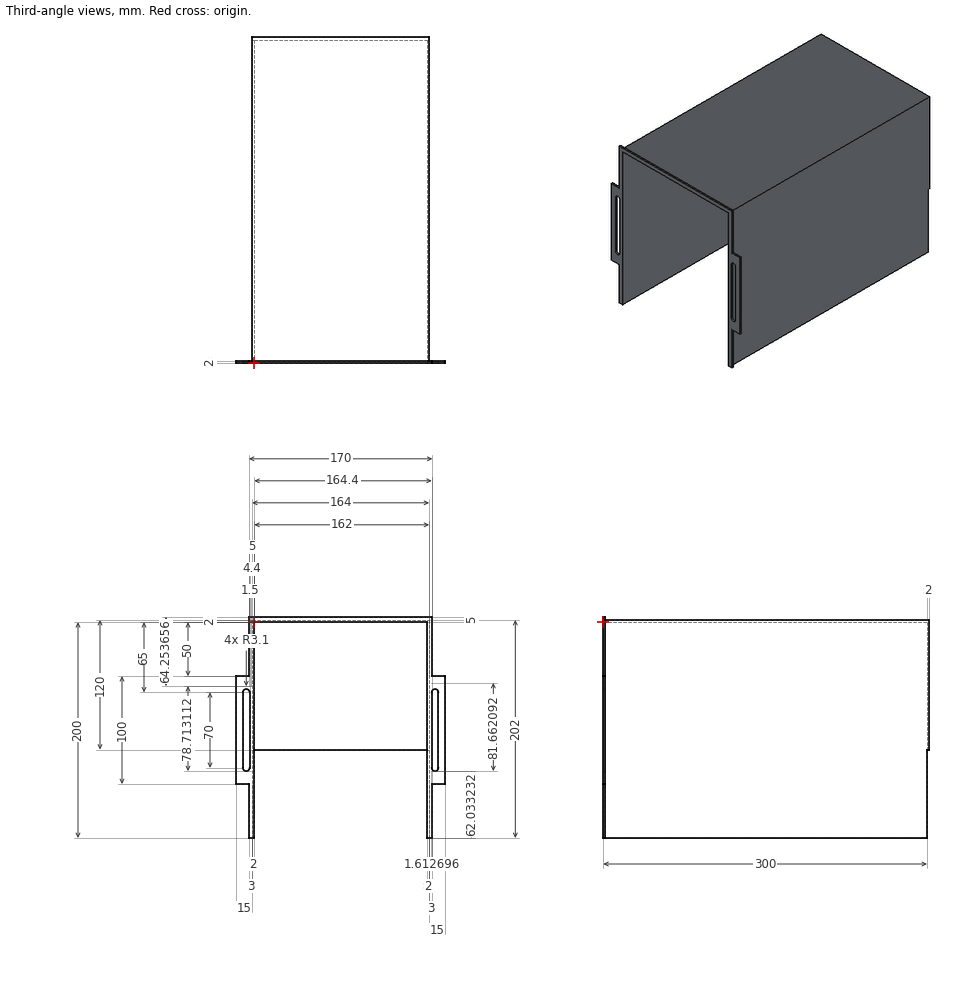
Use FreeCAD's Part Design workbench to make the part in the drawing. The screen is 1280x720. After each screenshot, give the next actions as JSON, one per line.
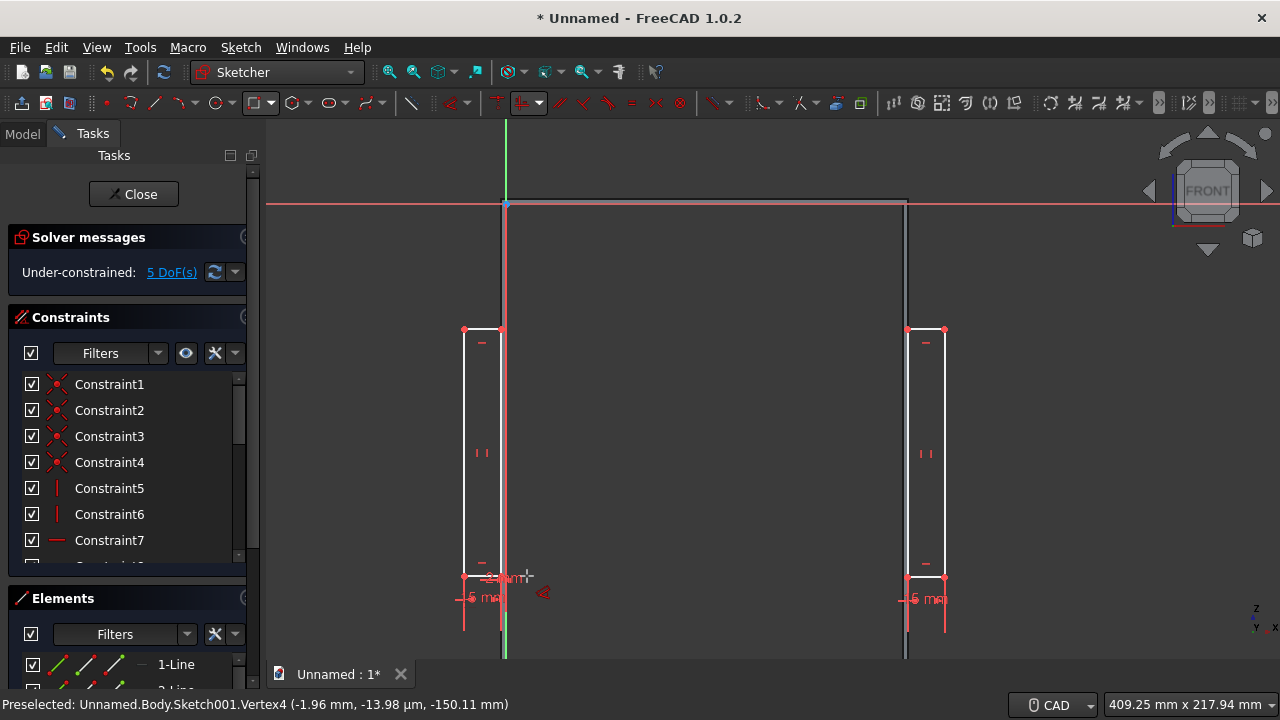
{"action": "left_click", "coordinate": [464, 404]}
{"action": "left_click", "coordinate": [430, 453]}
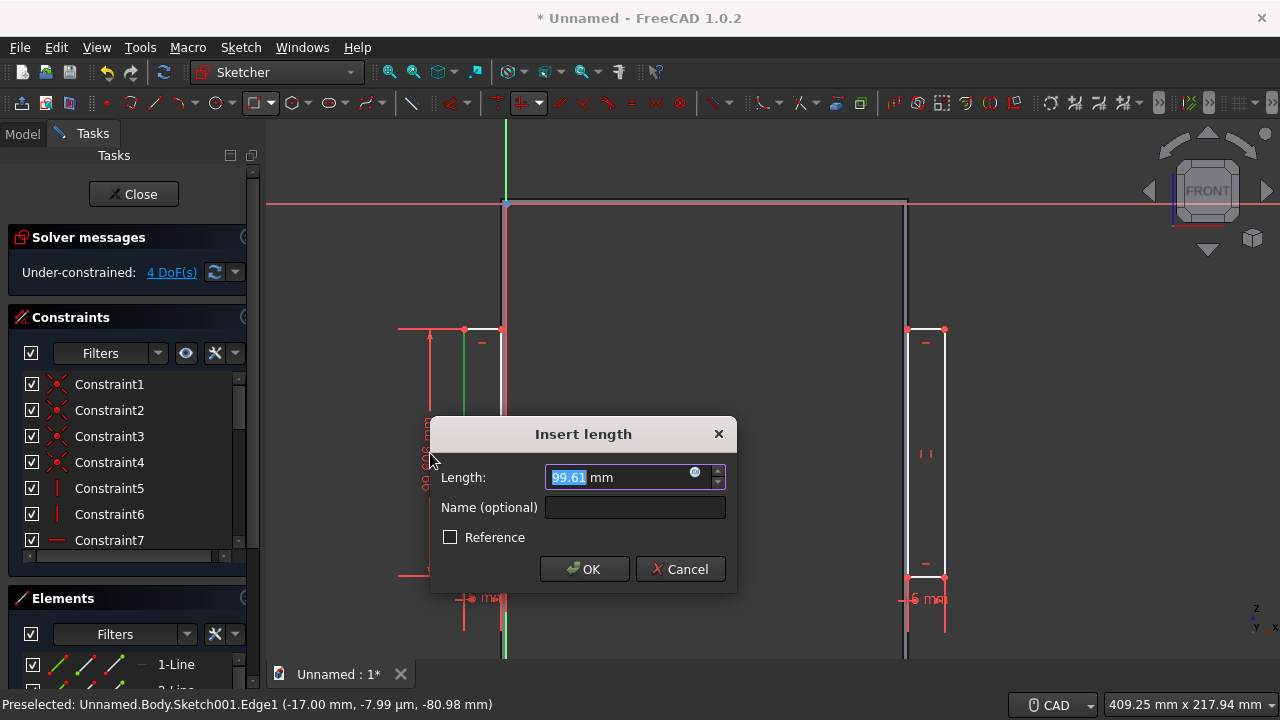
{"action": "type", "text": "100"}
{"action": "key", "text": "Return"}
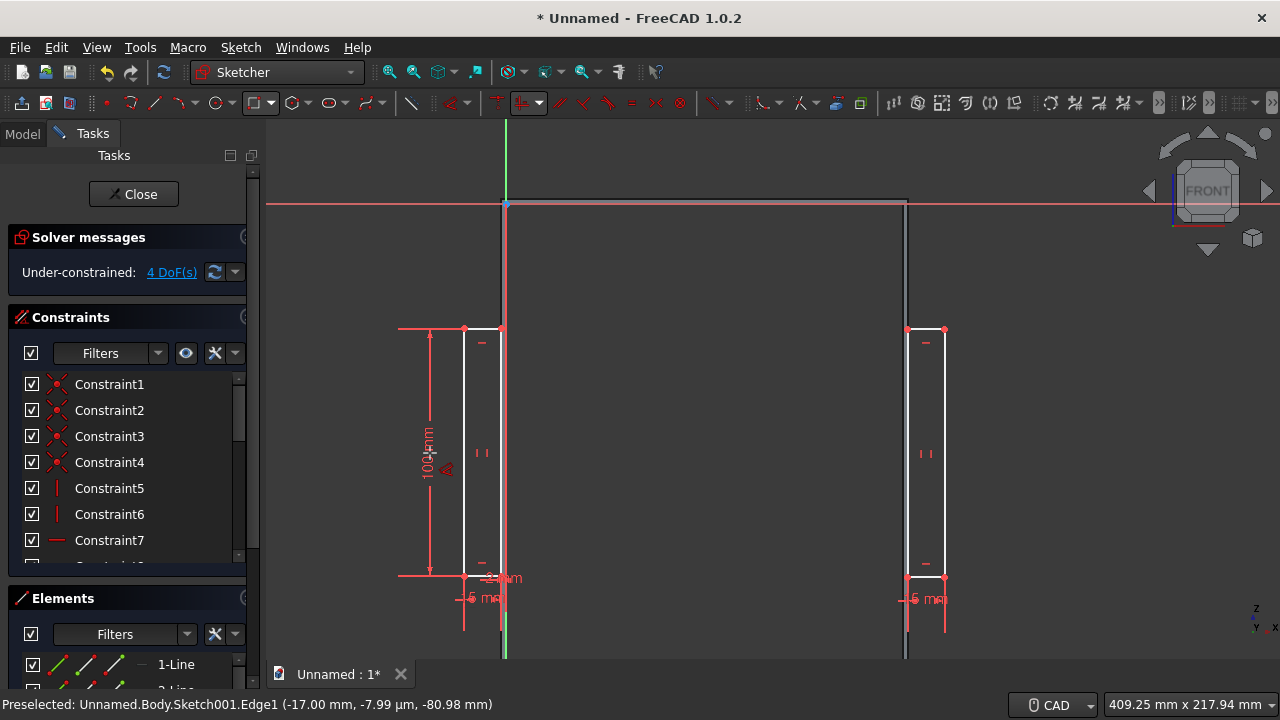
{"action": "left_click", "coordinate": [908, 404]}
{"action": "left_click", "coordinate": [874, 453]}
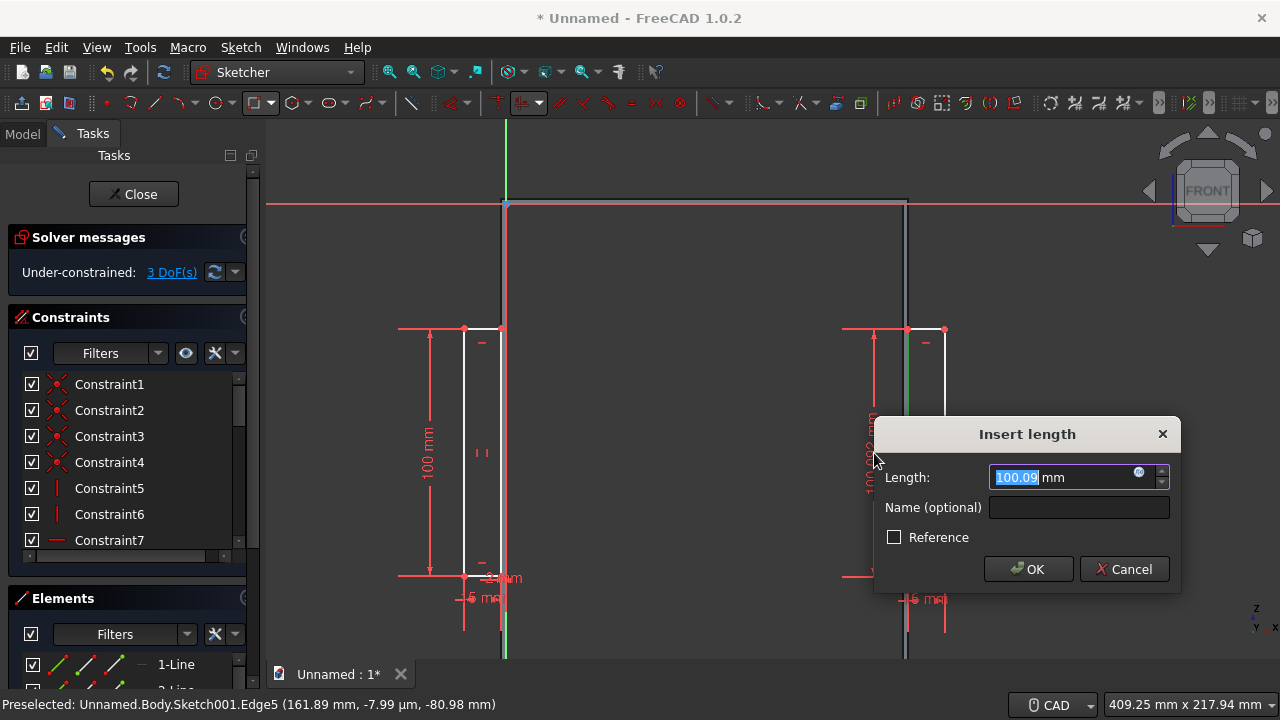
{"action": "type", "text": "100"}
{"action": "key", "text": "Return"}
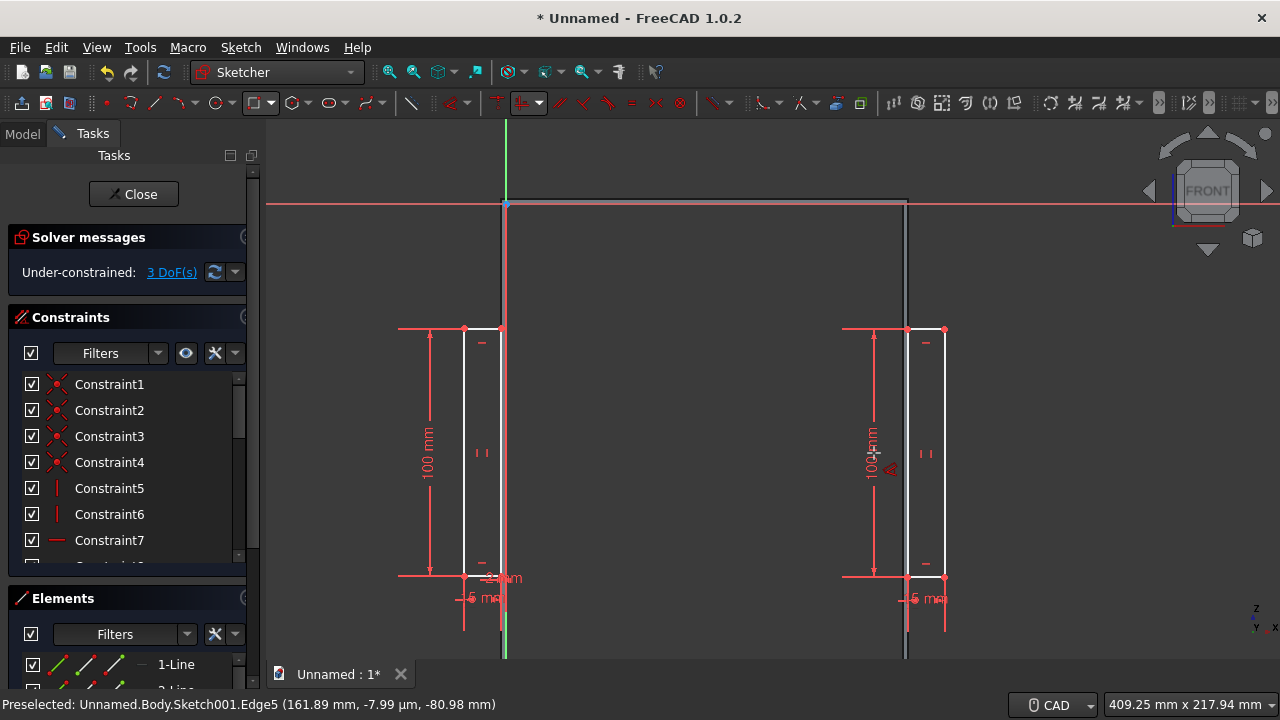
{"action": "left_click", "coordinate": [464, 329]}
{"action": "left_click", "coordinate": [430, 267]}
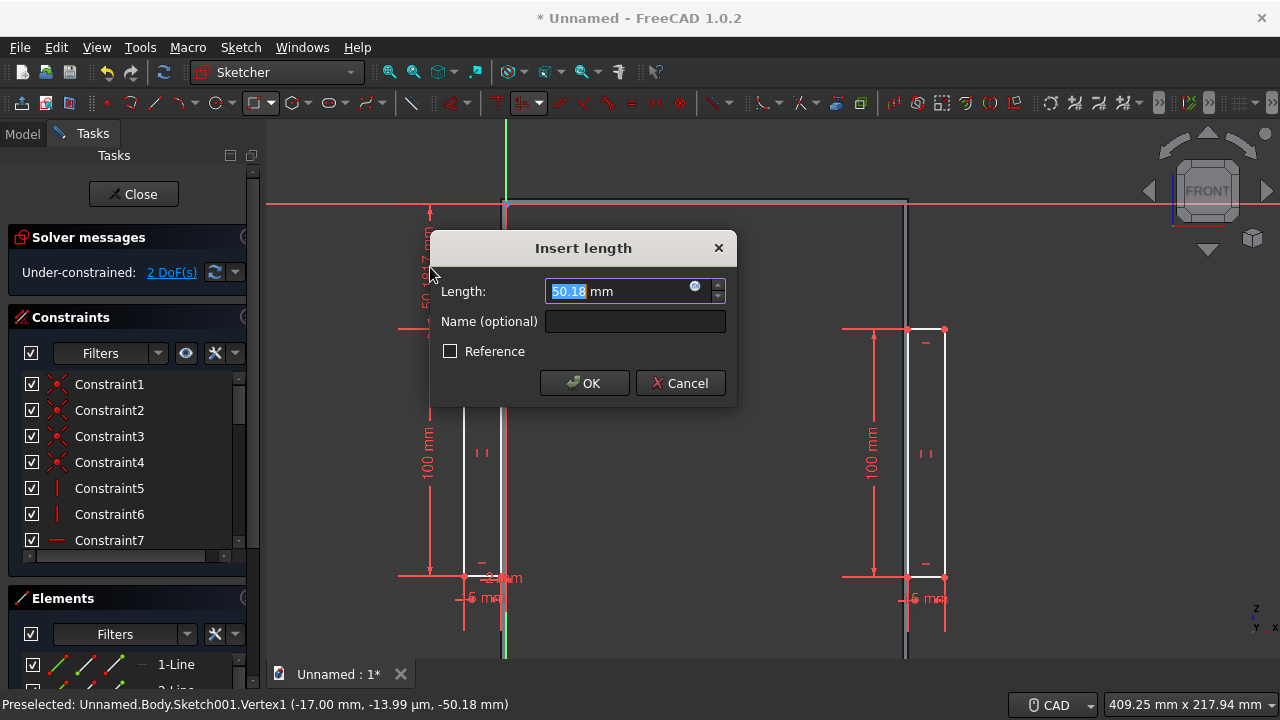
{"action": "type", "text": "50"}
{"action": "key", "text": "Return"}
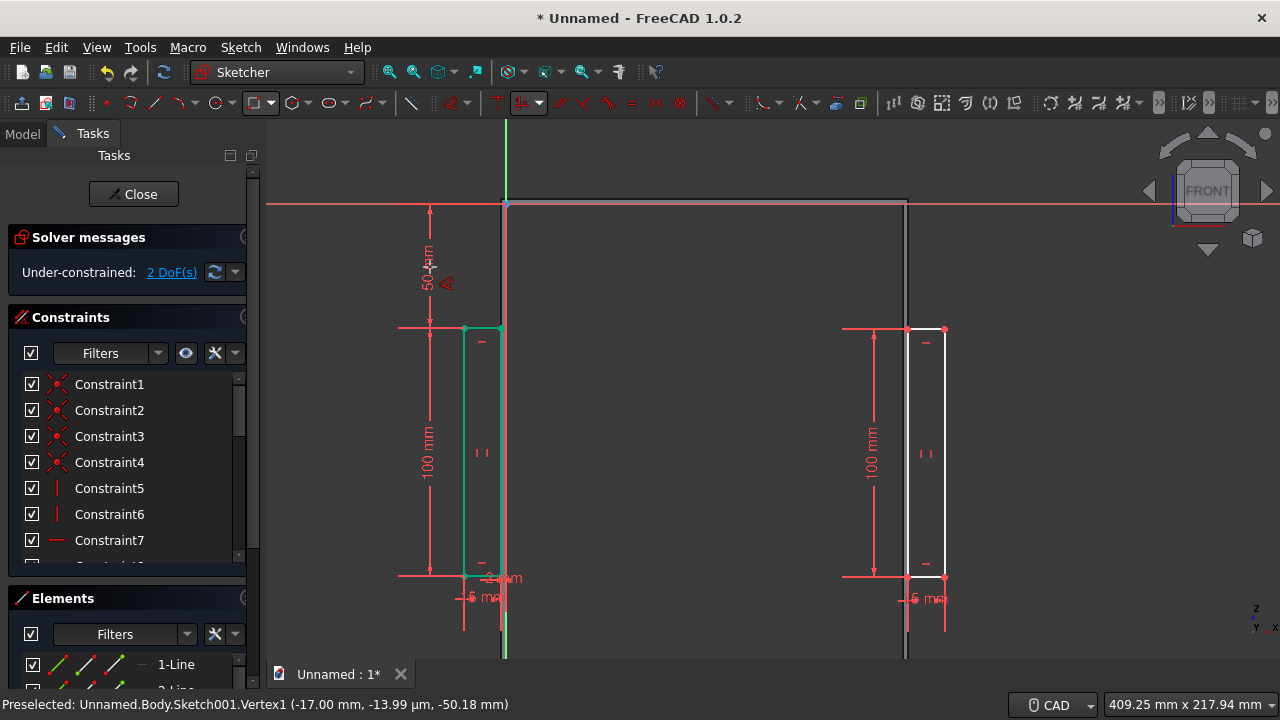
{"action": "left_click", "coordinate": [908, 329]}
{"action": "left_click", "coordinate": [942, 267]}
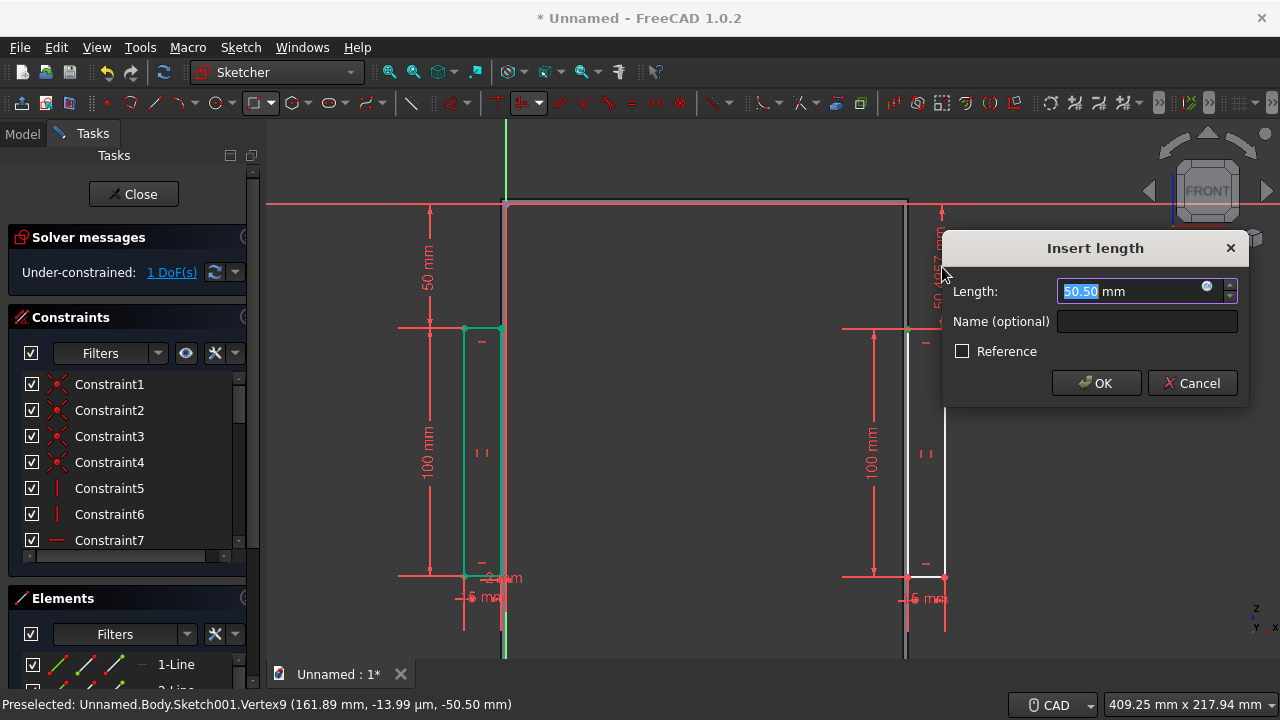
{"action": "type", "text": "50"}
{"action": "key", "text": "Return"}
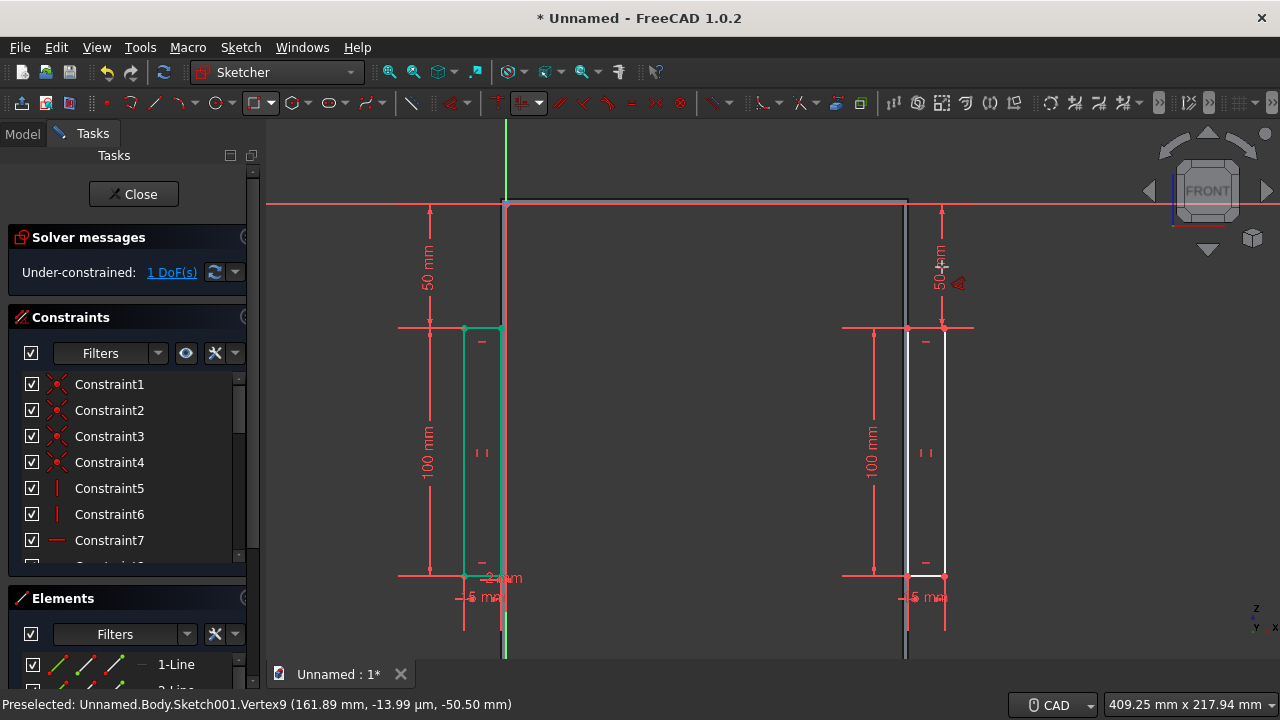
{"action": "left_click", "coordinate": [908, 328]}
{"action": "left_click", "coordinate": [707, 170]}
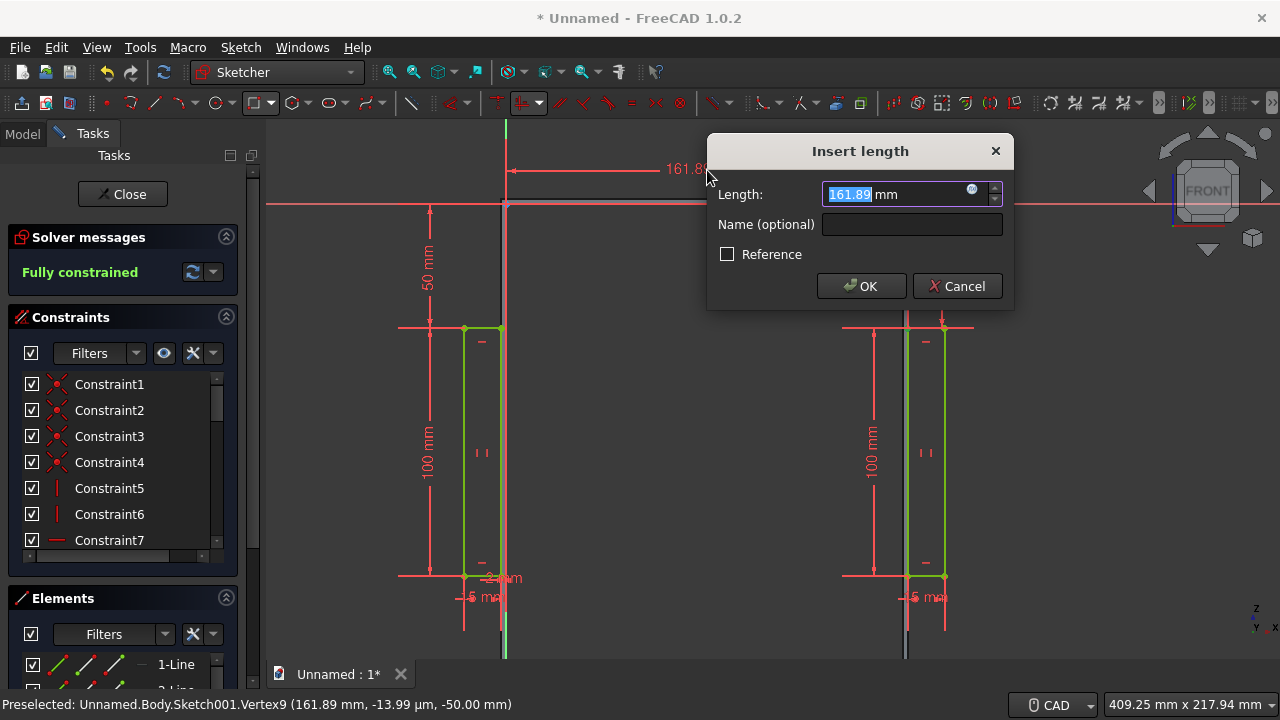
{"action": "type", "text": "162"}
{"action": "key", "text": "Return"}
{"action": "key", "text": "Escape"}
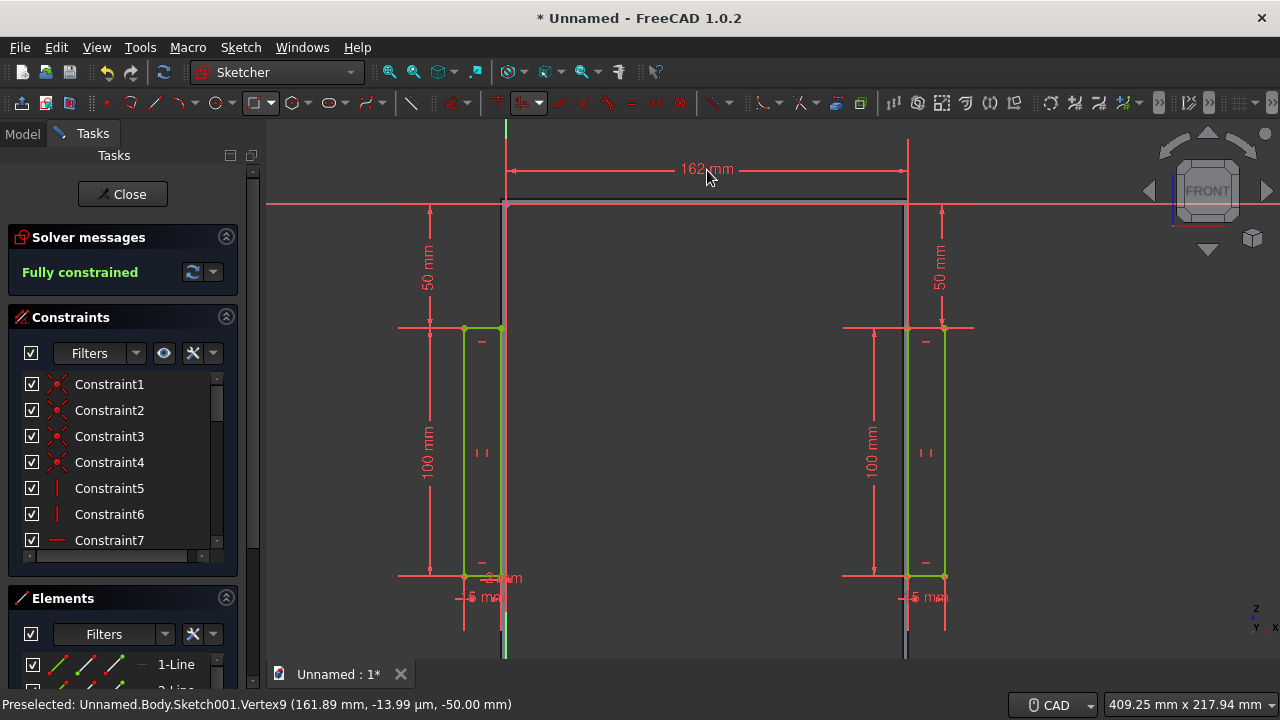
{"action": "left_click", "coordinate": [123, 194]}